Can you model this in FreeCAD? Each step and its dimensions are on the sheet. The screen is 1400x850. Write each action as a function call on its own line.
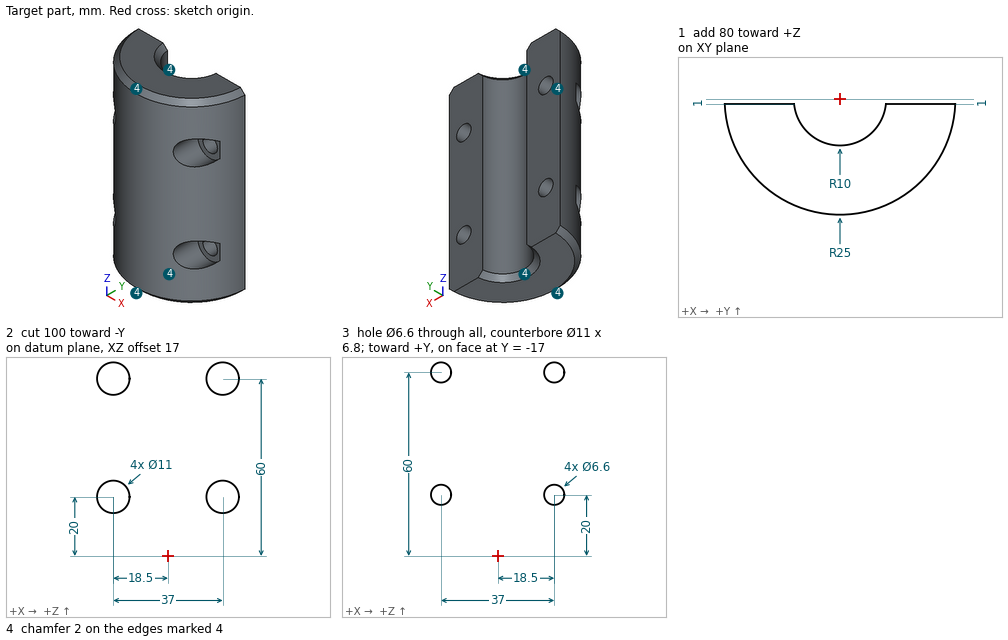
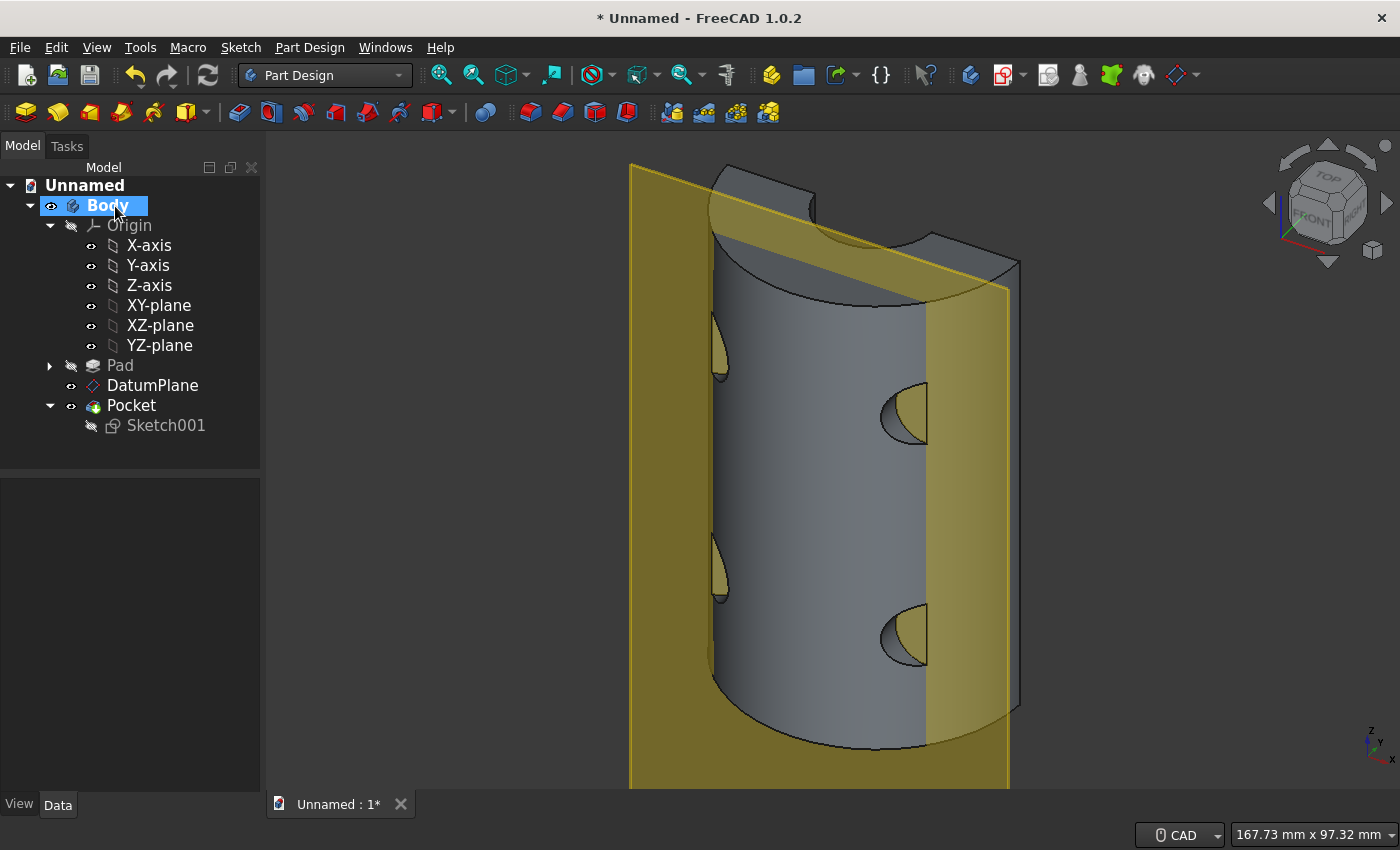
click(116, 386)
key(space)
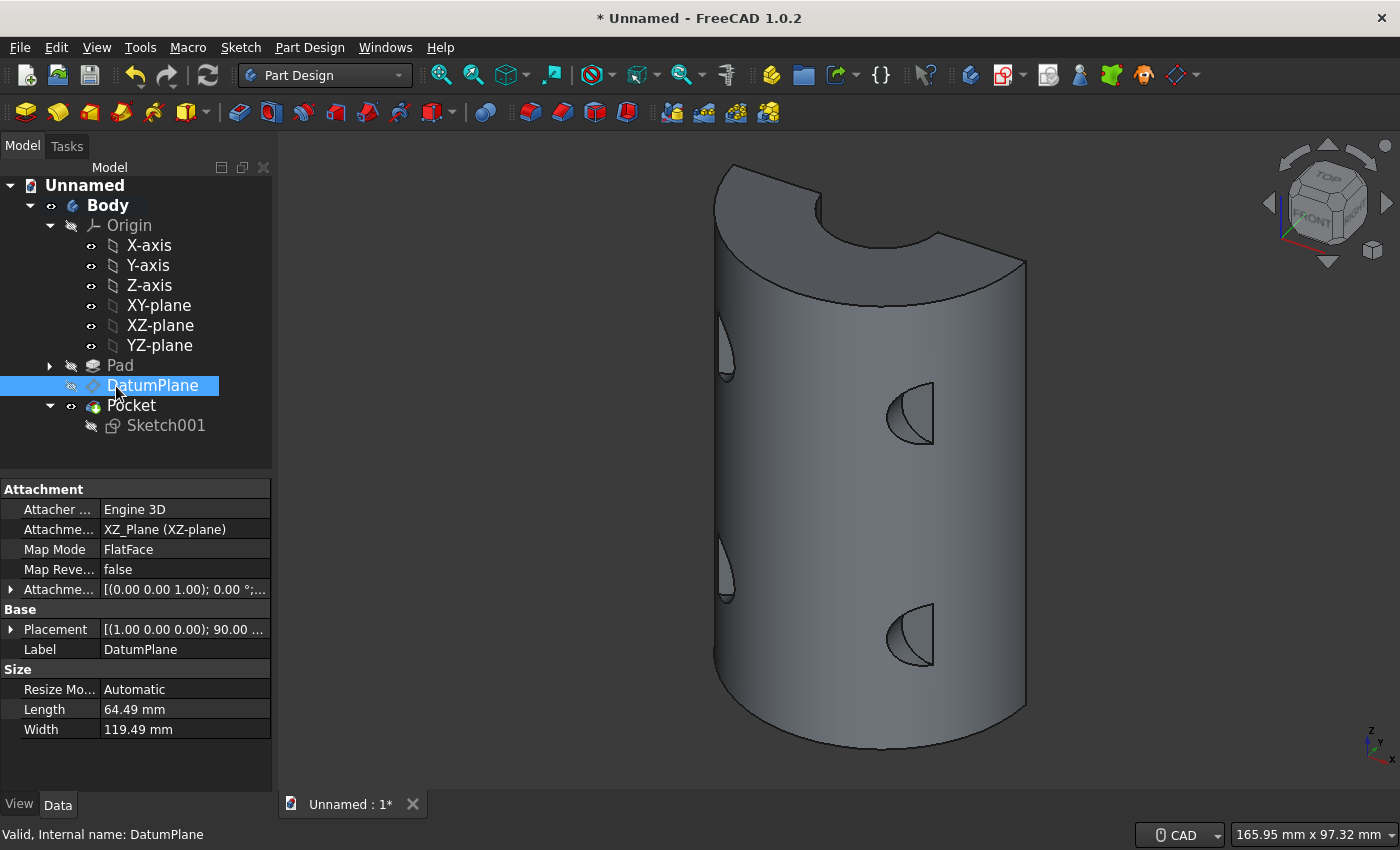
key(0)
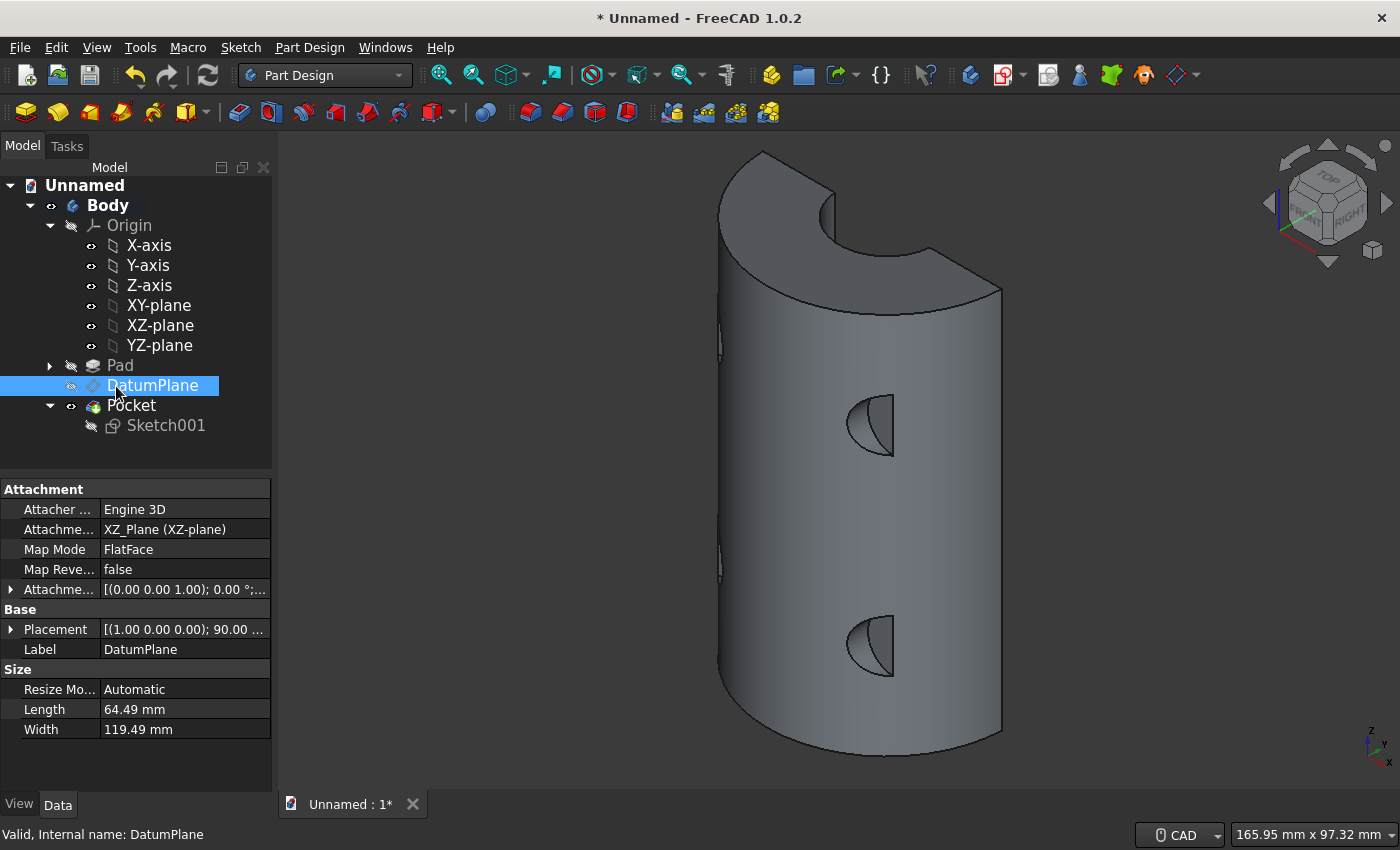
click(442, 76)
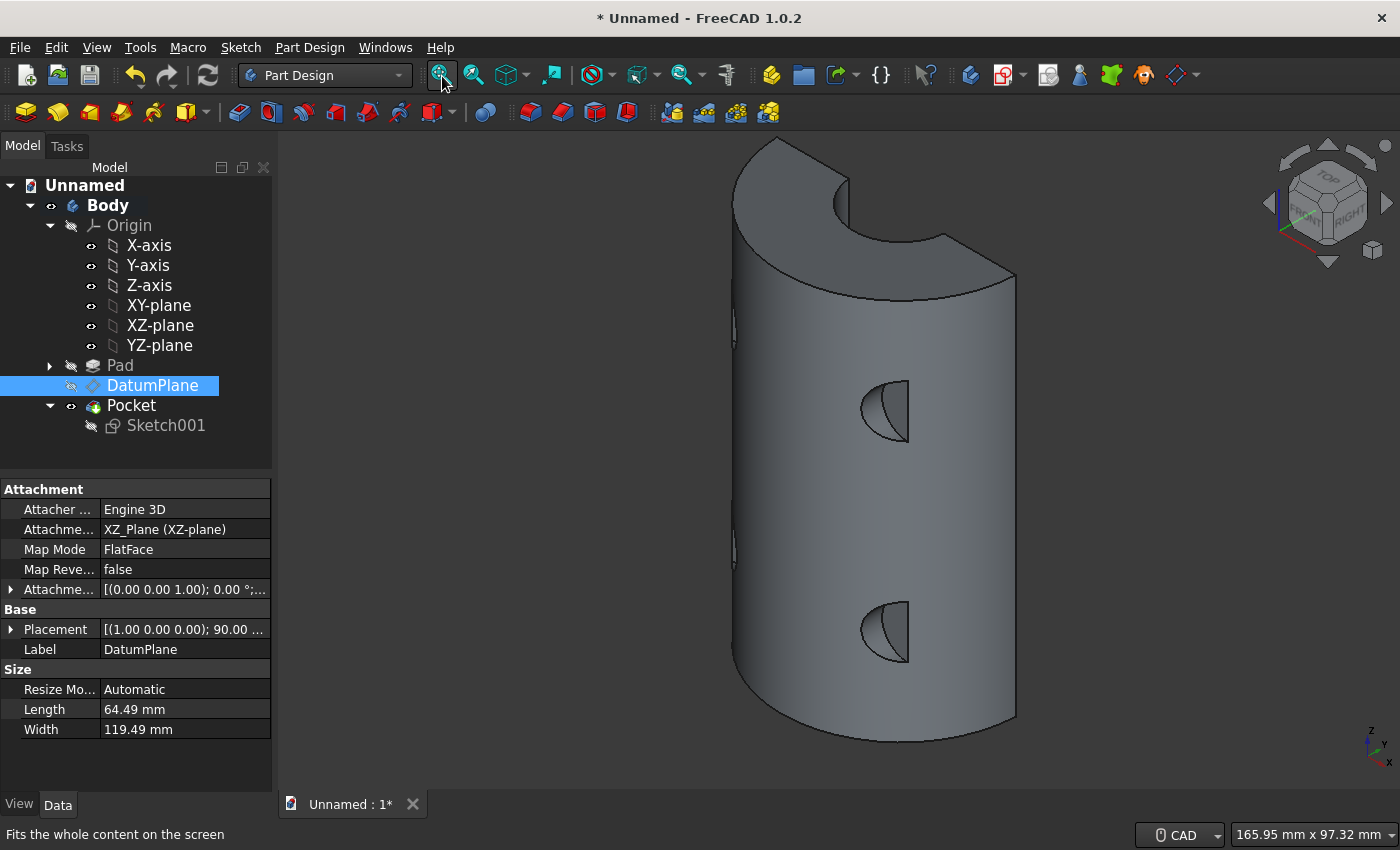
key(1)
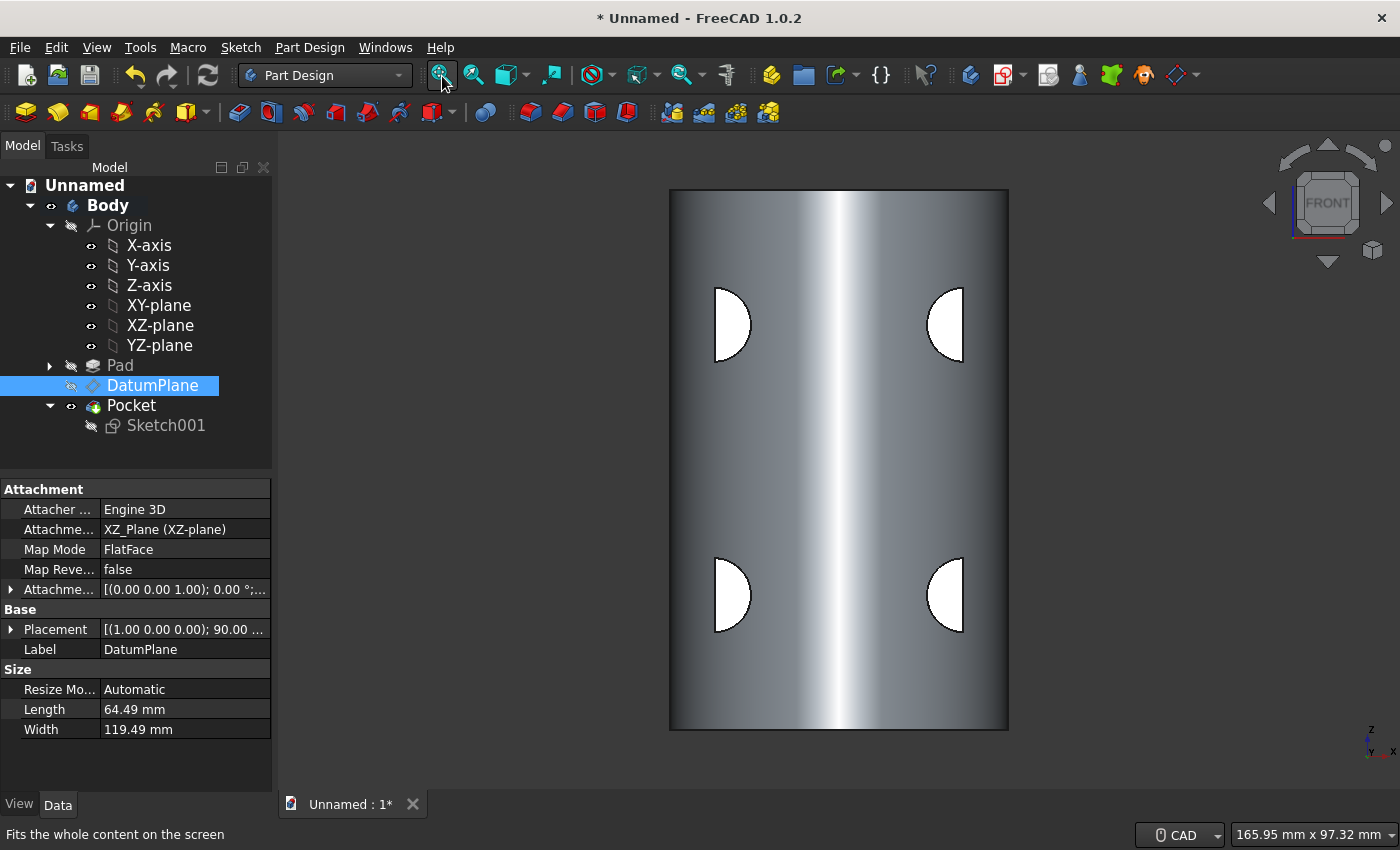
click(733, 324)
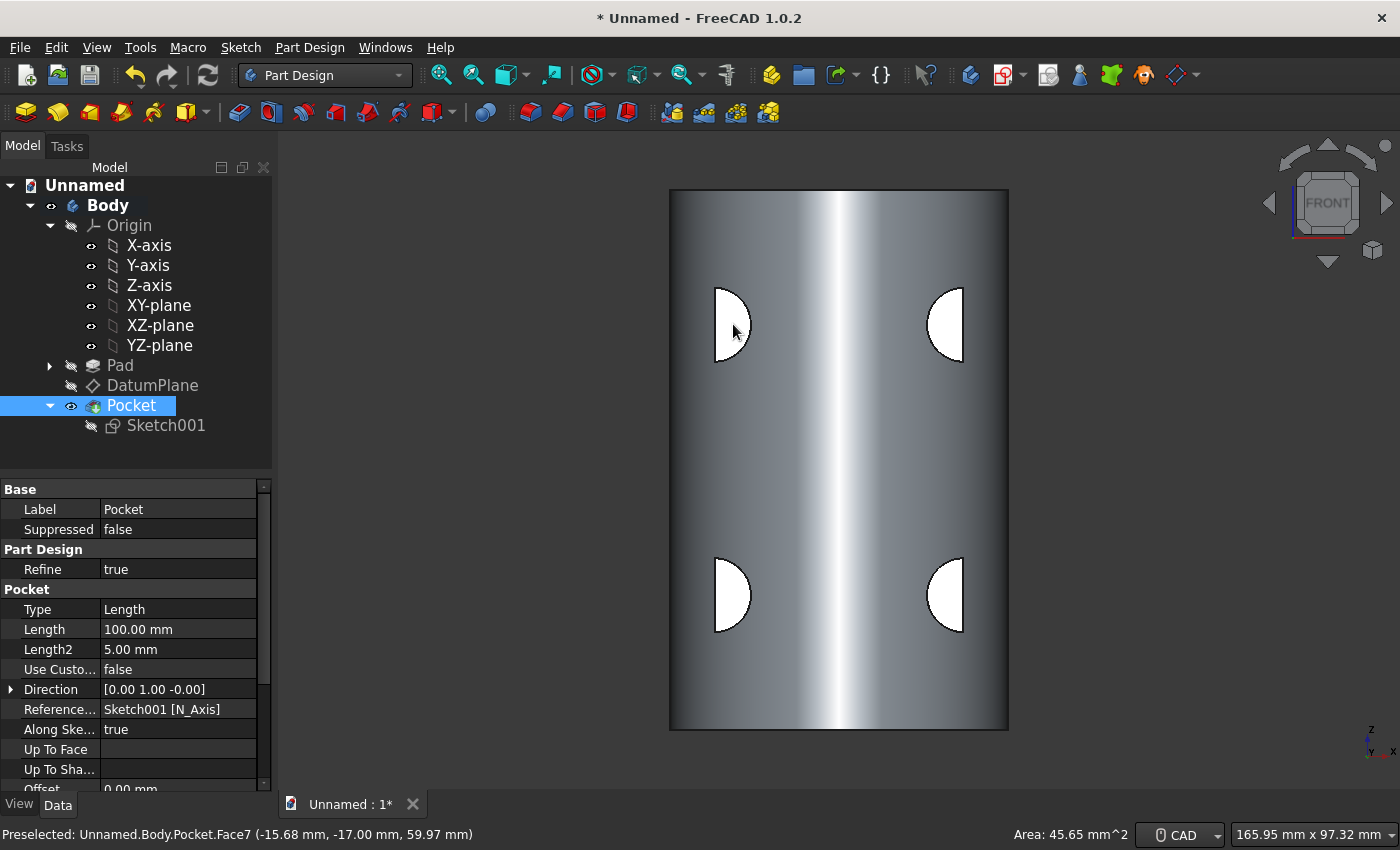
click(1004, 76)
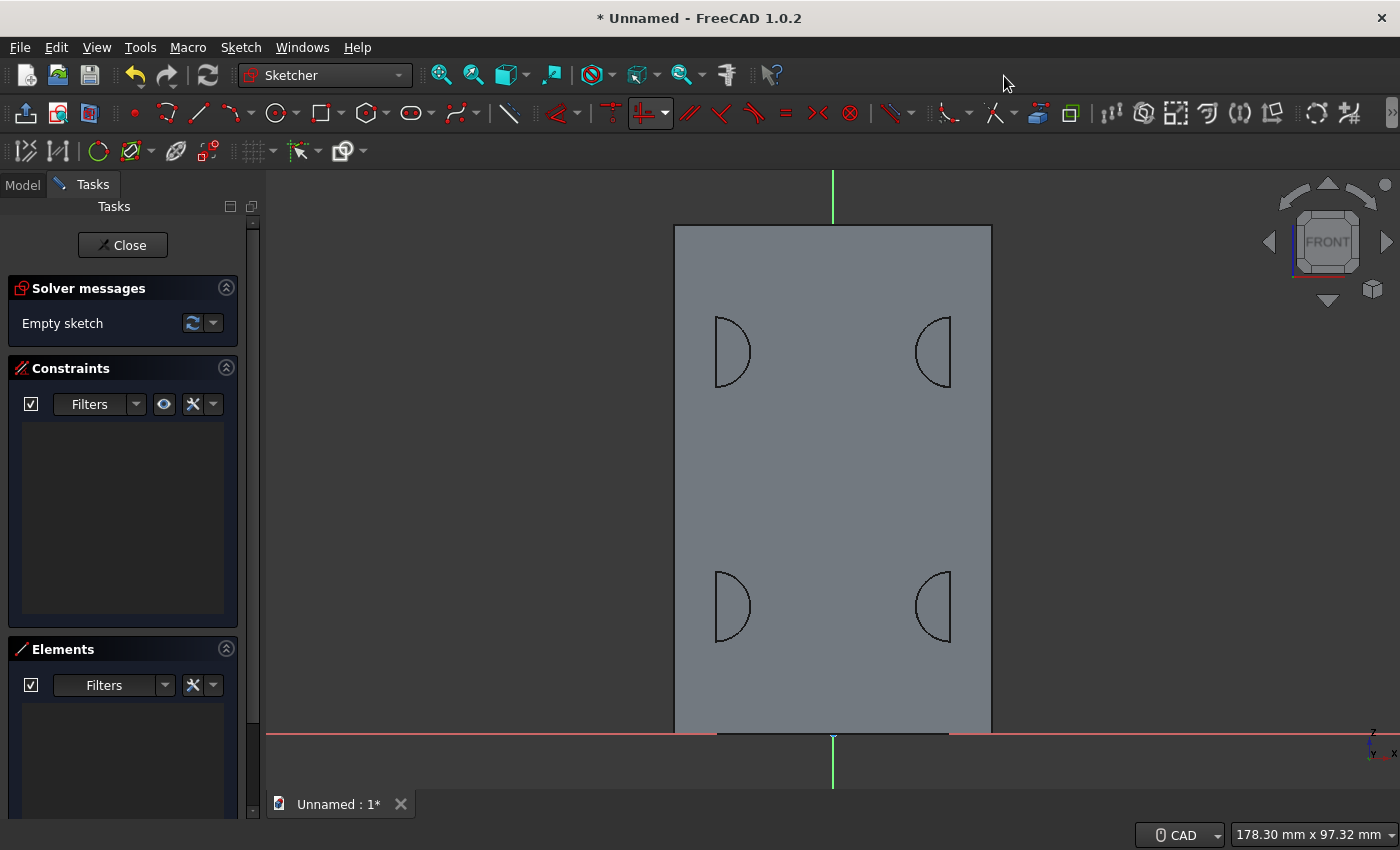
click(276, 114)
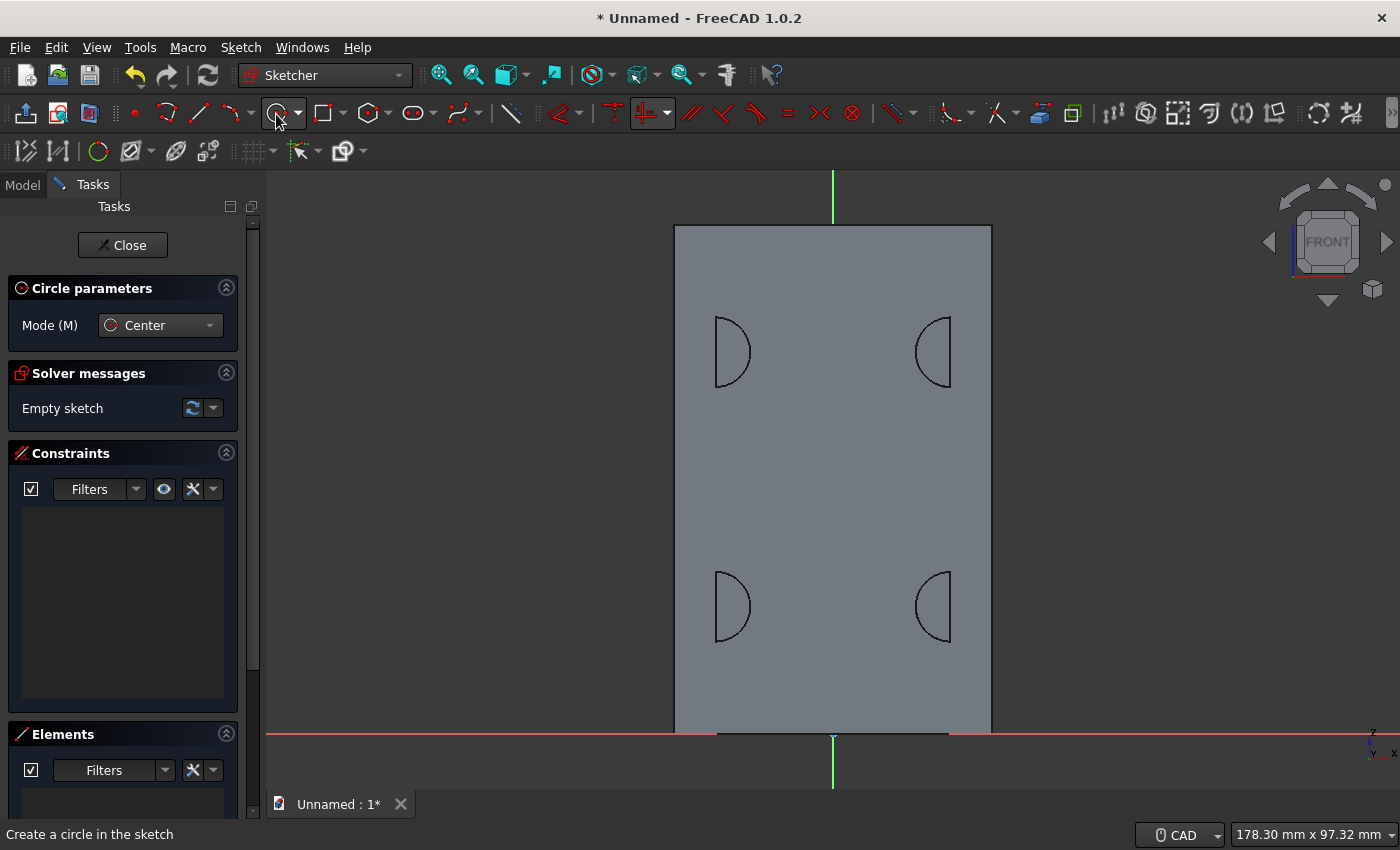
click(951, 607)
move(966, 592)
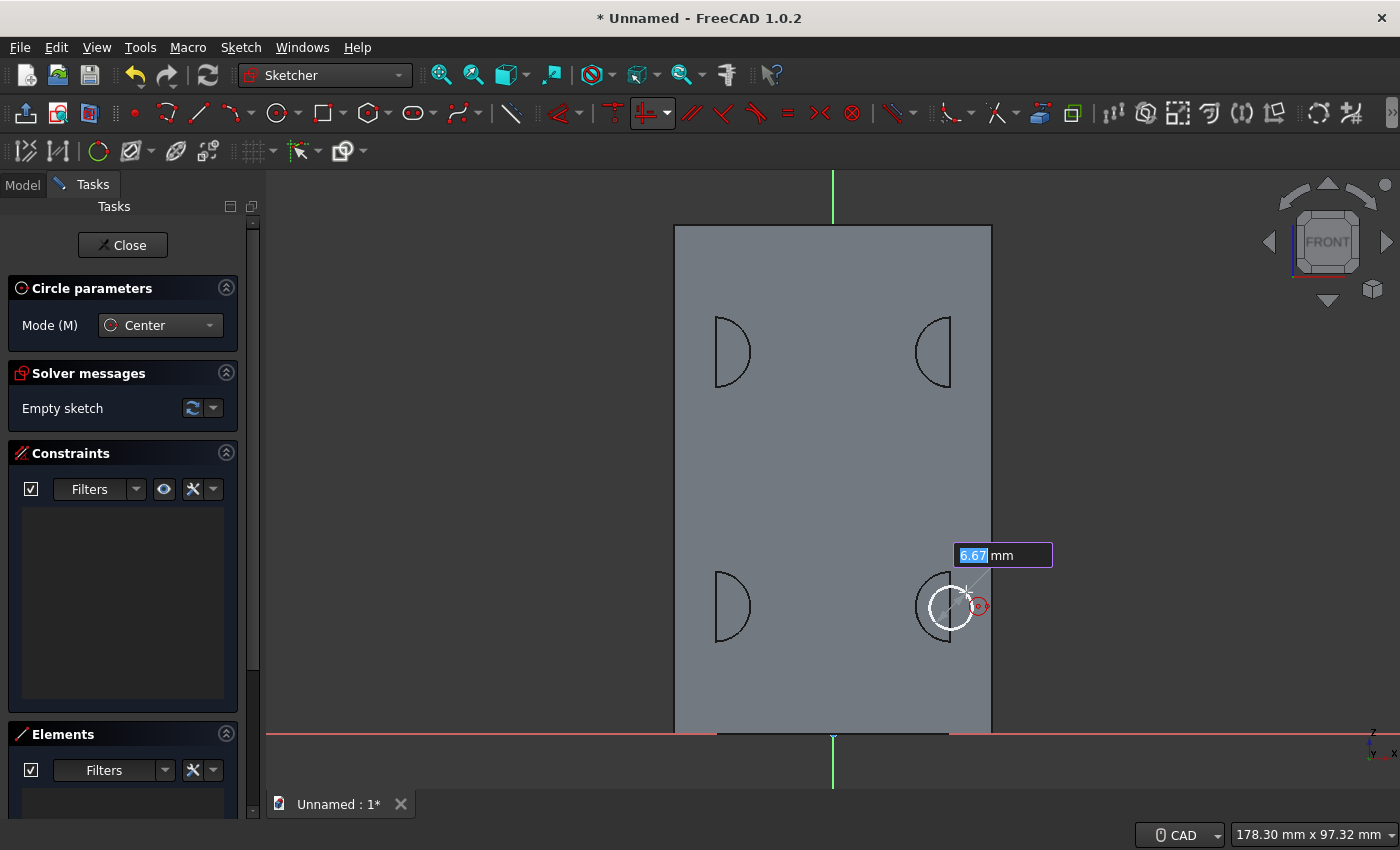
text(6.6)
key(Return)